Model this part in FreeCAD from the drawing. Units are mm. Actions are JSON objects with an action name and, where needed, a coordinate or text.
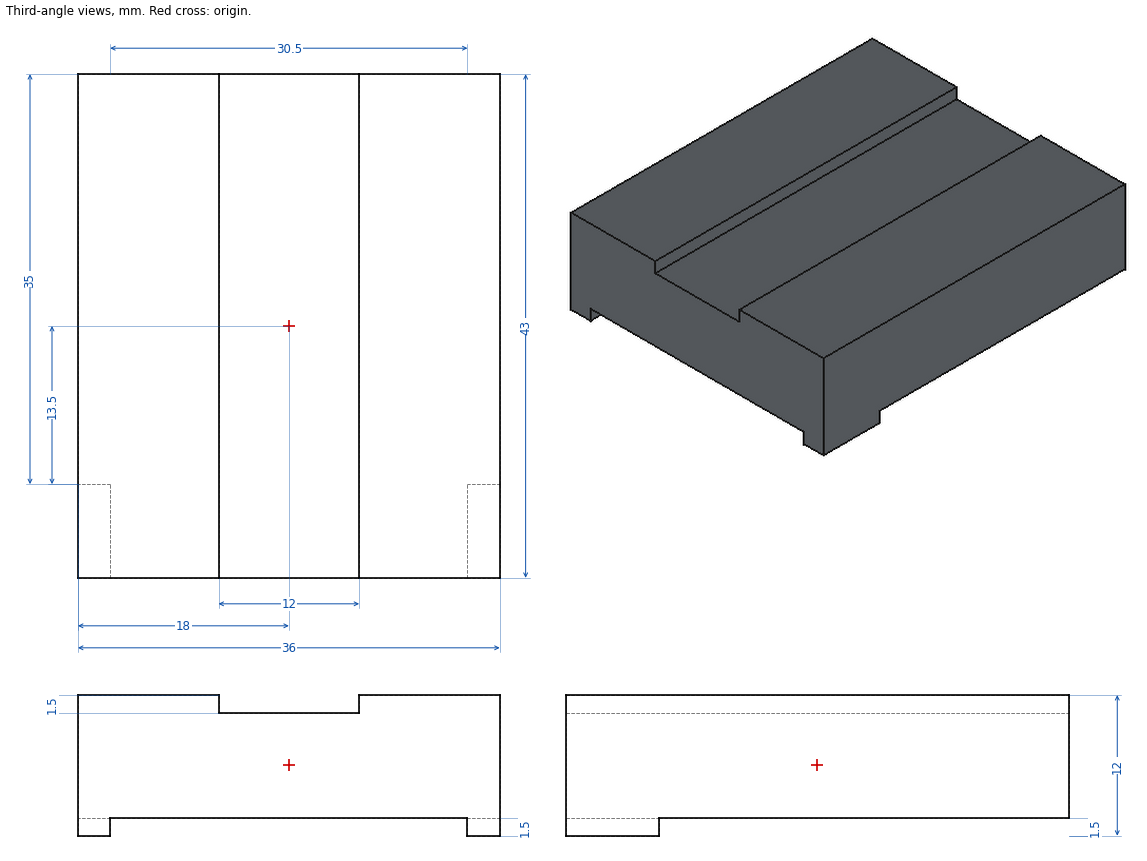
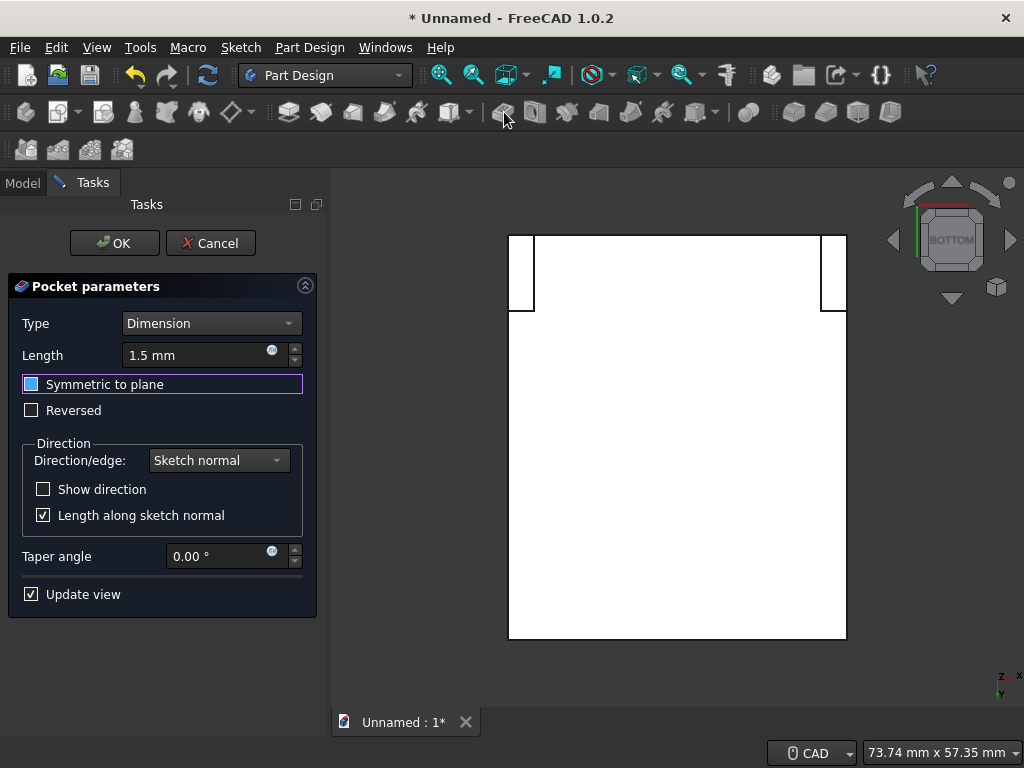
{"action": "left_click", "coordinate": [115, 243]}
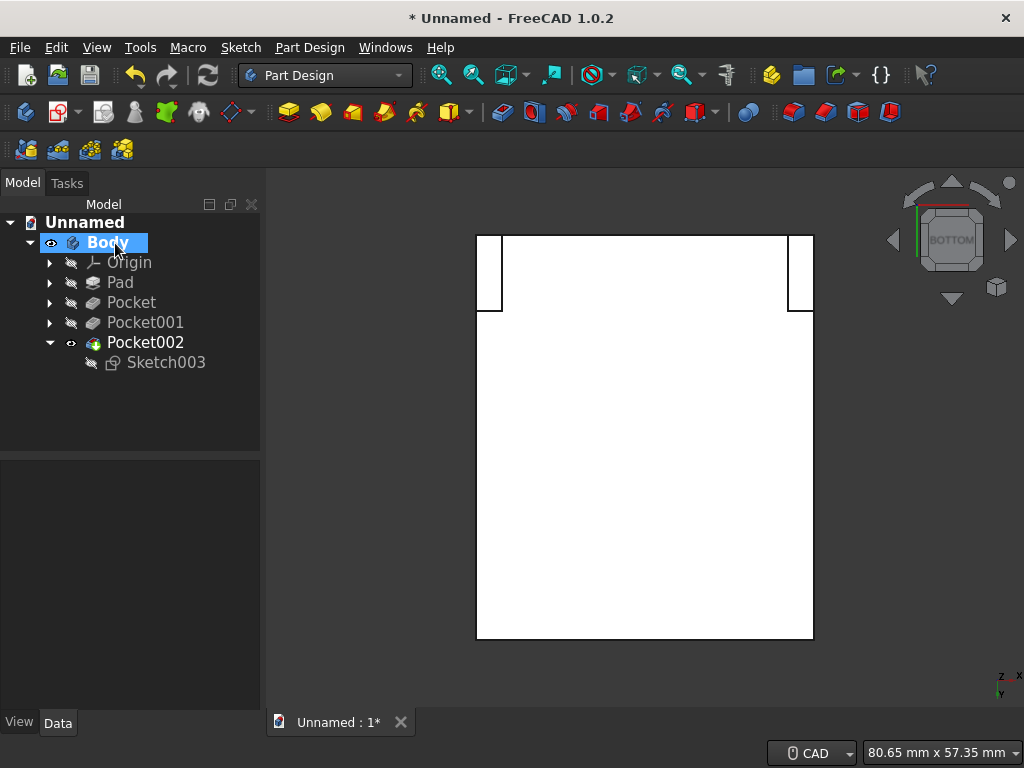
{"action": "key", "text": "0"}